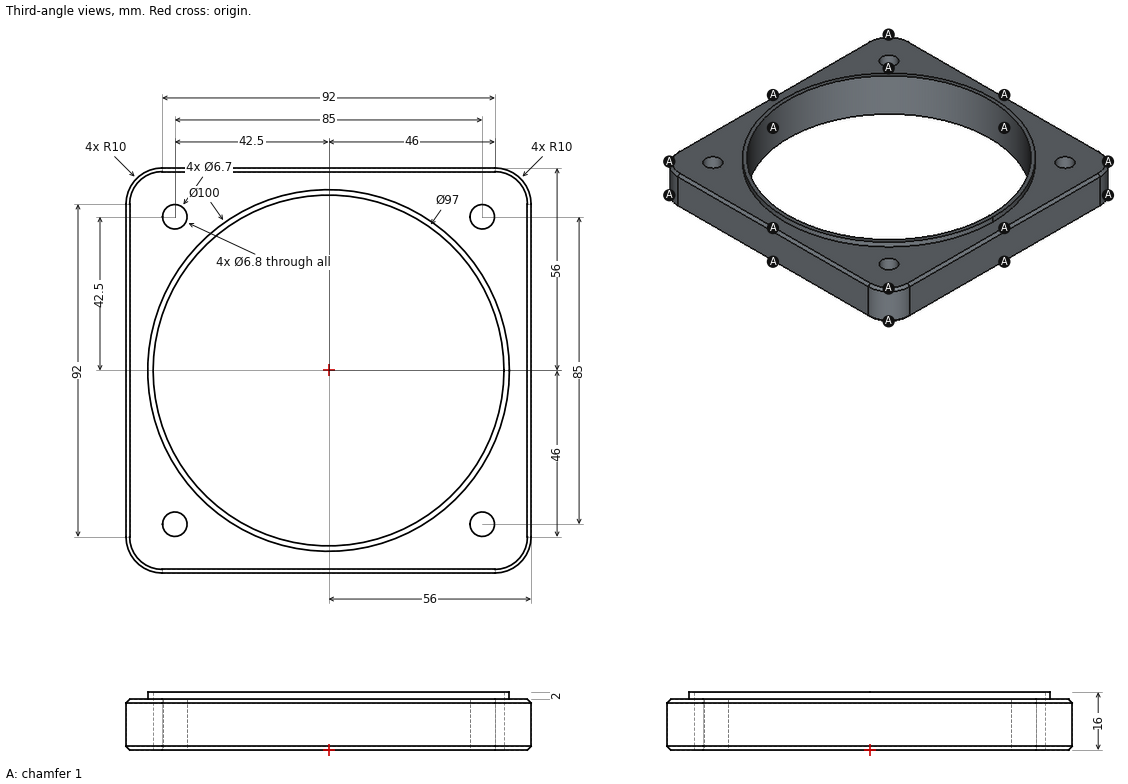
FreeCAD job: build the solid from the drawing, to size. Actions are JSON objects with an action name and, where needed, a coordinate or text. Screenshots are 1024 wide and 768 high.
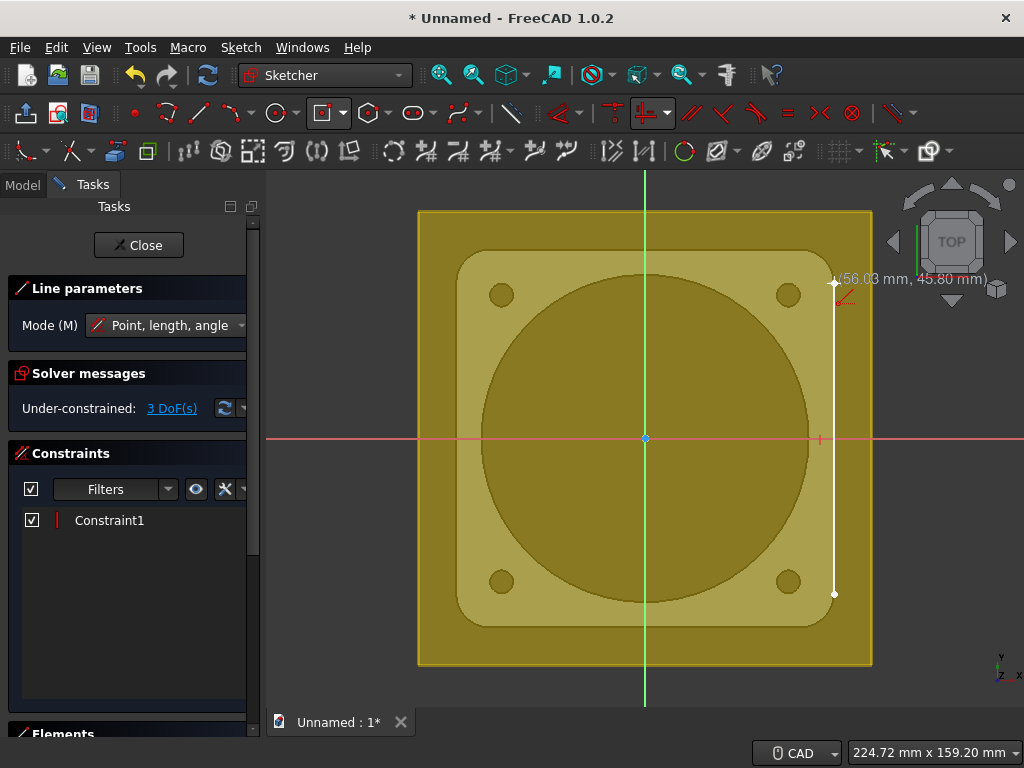
{"action": "left_click", "coordinate": [800, 250]}
{"action": "left_click", "coordinate": [490, 250]}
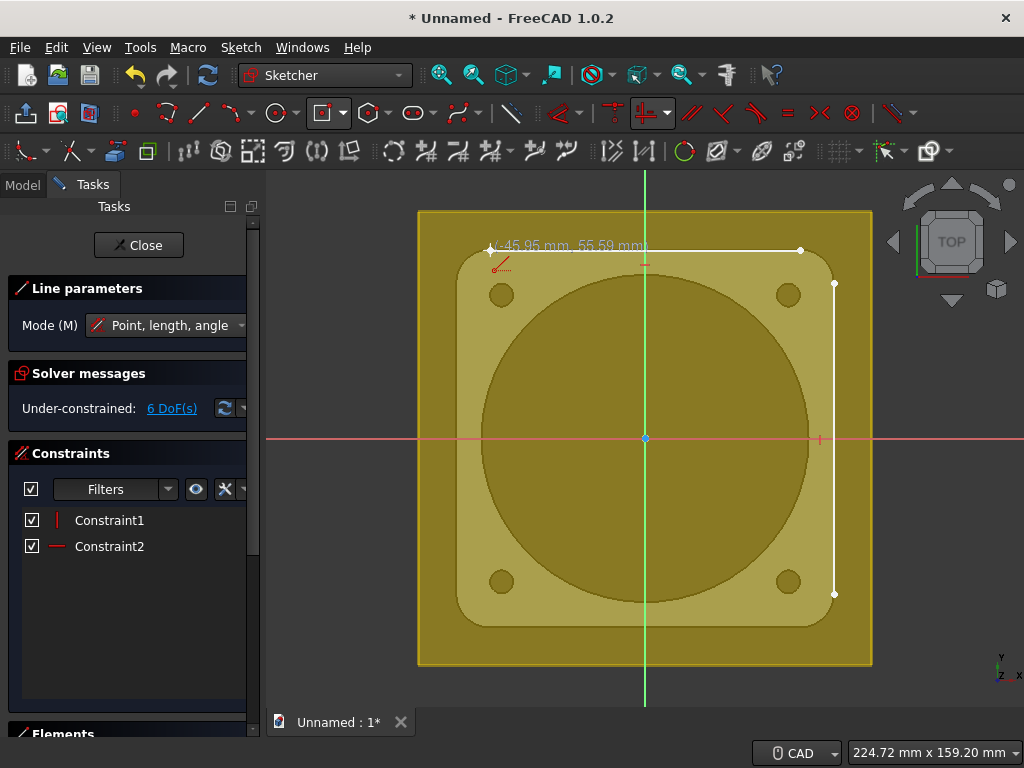
{"action": "left_click", "coordinate": [456, 283]}
{"action": "left_click", "coordinate": [456, 594]}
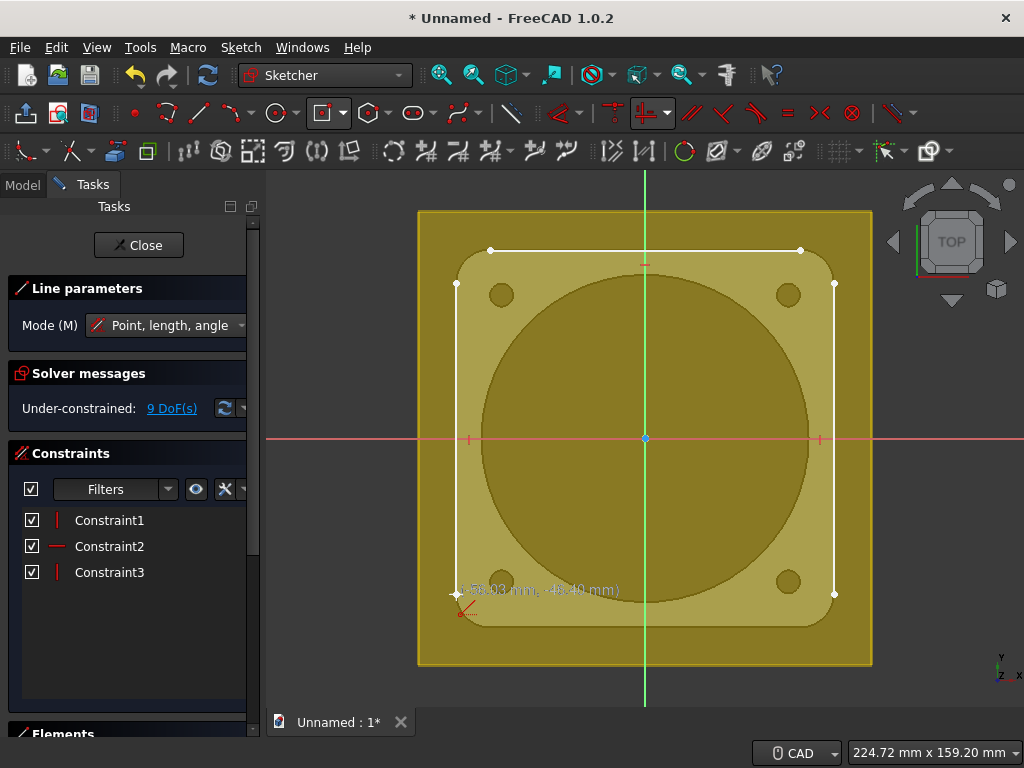
{"action": "left_click", "coordinate": [490, 627]}
{"action": "left_click", "coordinate": [800, 627]}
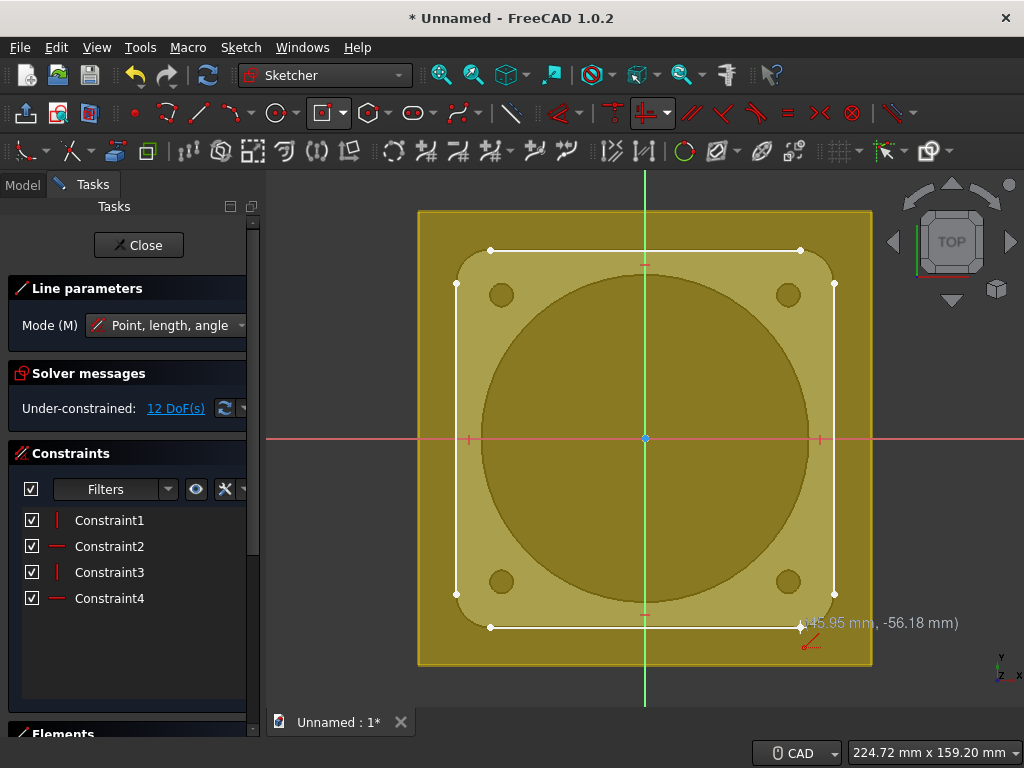
{"action": "left_click", "coordinate": [232, 114]}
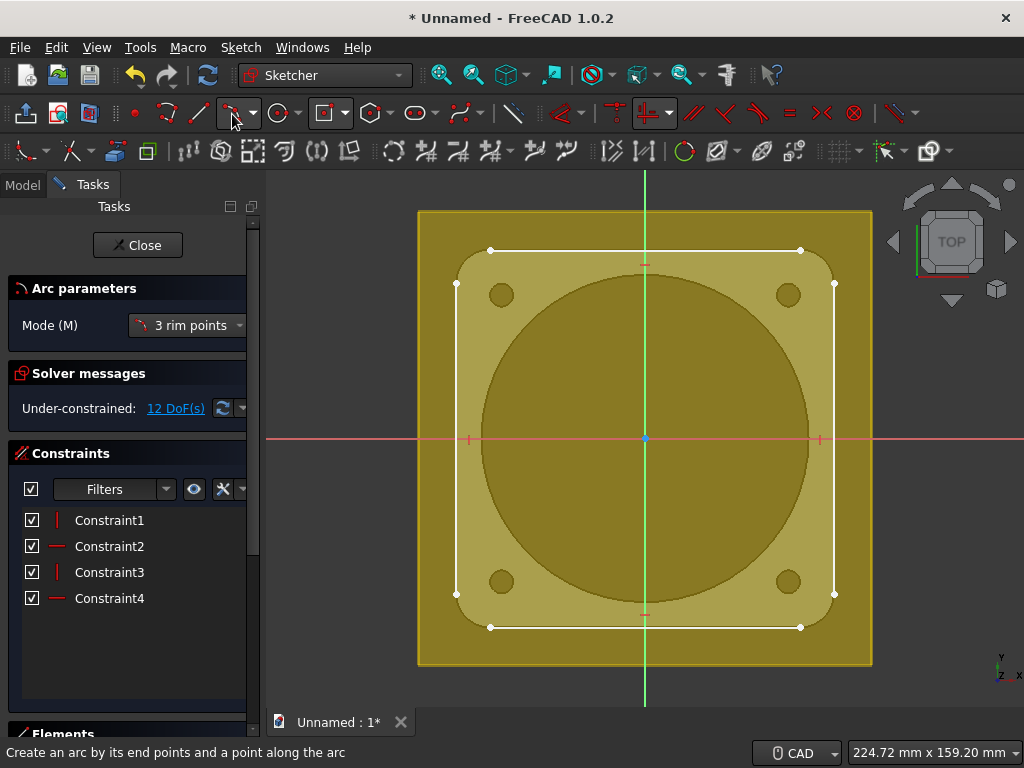
{"action": "left_click", "coordinate": [834, 284]}
{"action": "left_click", "coordinate": [800, 251]}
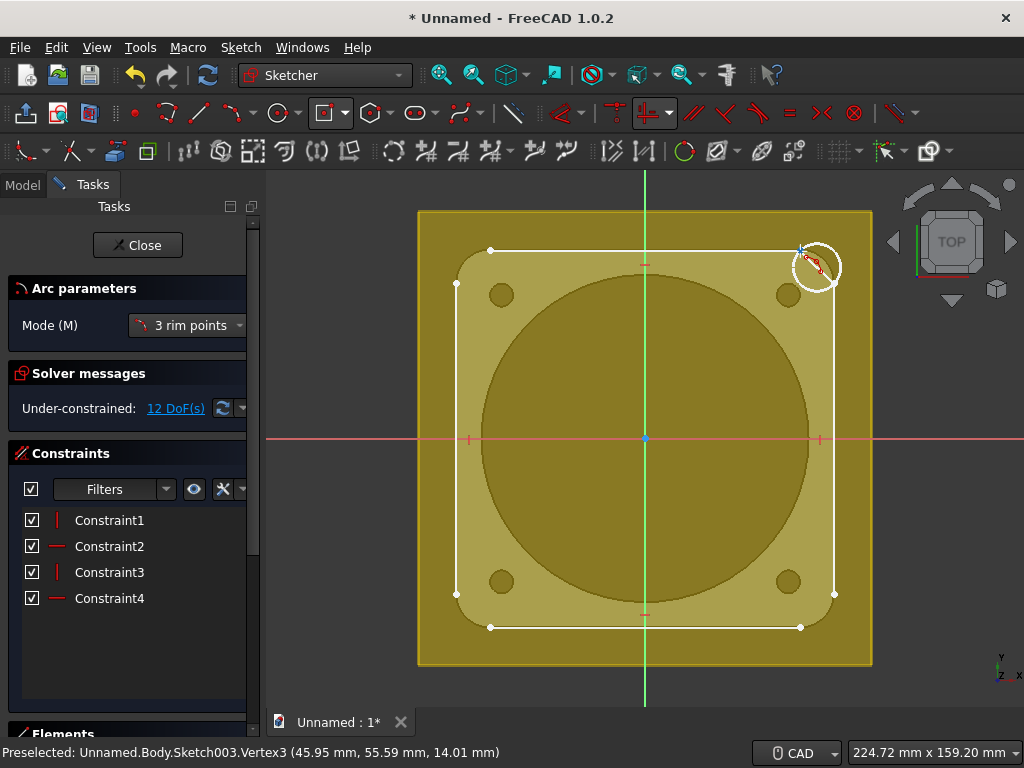
{"action": "scroll", "coordinate": [824, 259], "scroll_direction": "up", "scroll_amount": 3}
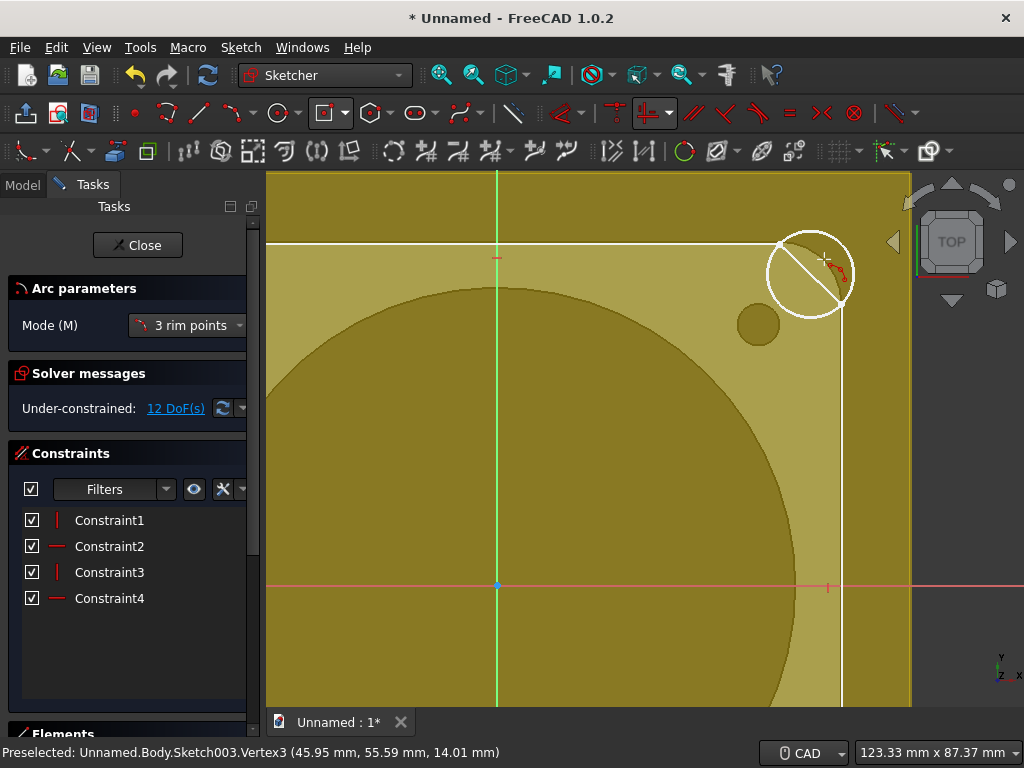
{"action": "left_click", "coordinate": [823, 260]}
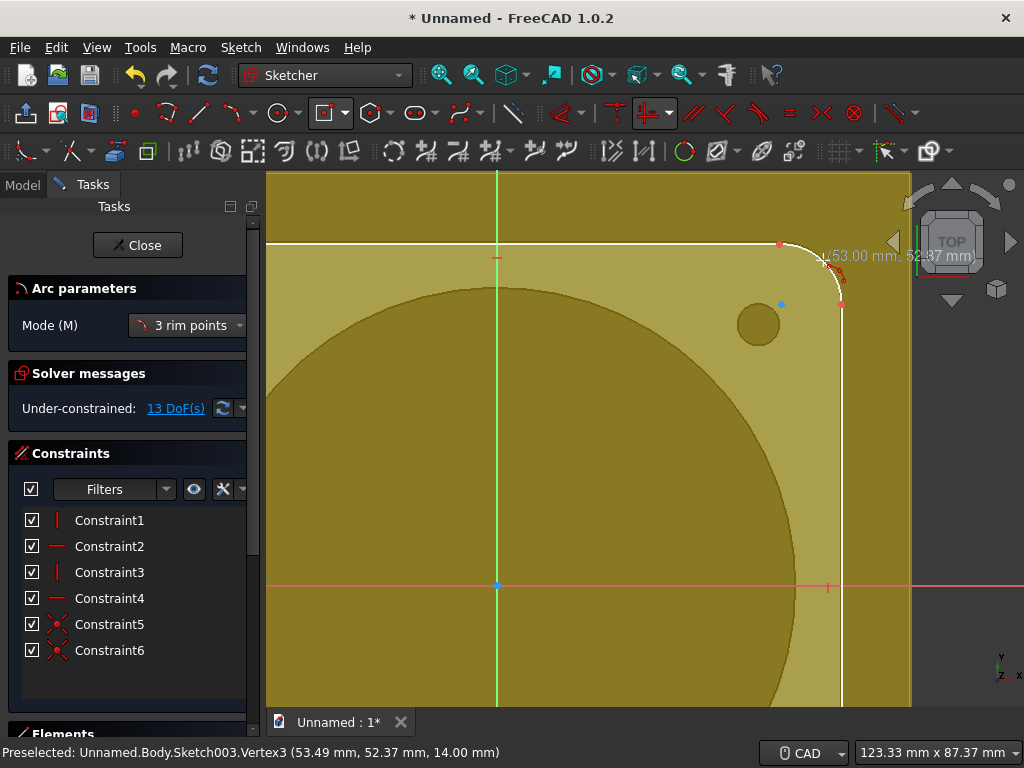
{"action": "scroll", "coordinate": [641, 318], "scroll_direction": "down", "scroll_amount": 4}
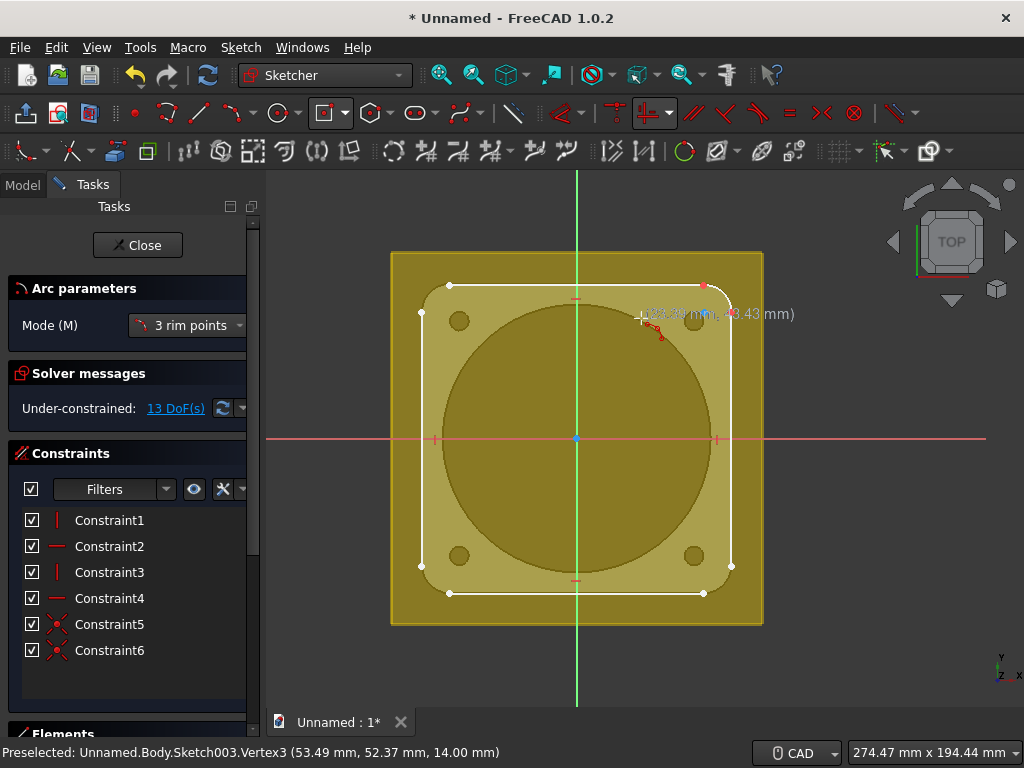
{"action": "left_click", "coordinate": [450, 285]}
{"action": "left_click", "coordinate": [422, 312]}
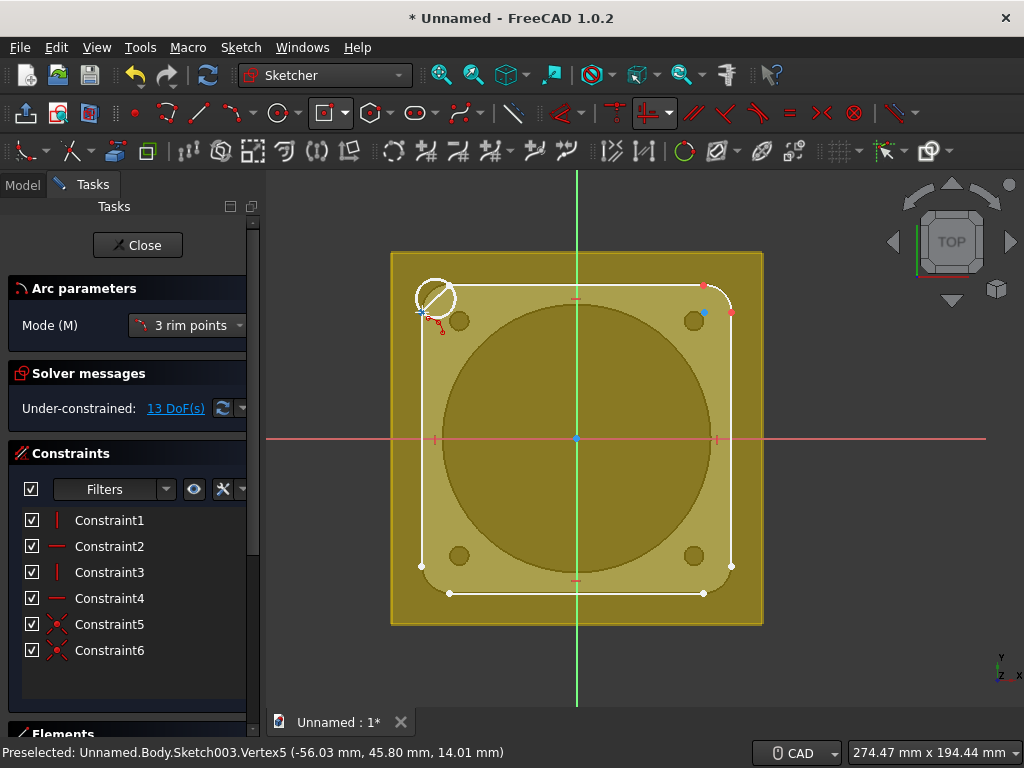
{"action": "scroll", "coordinate": [430, 292], "scroll_direction": "up", "scroll_amount": 4}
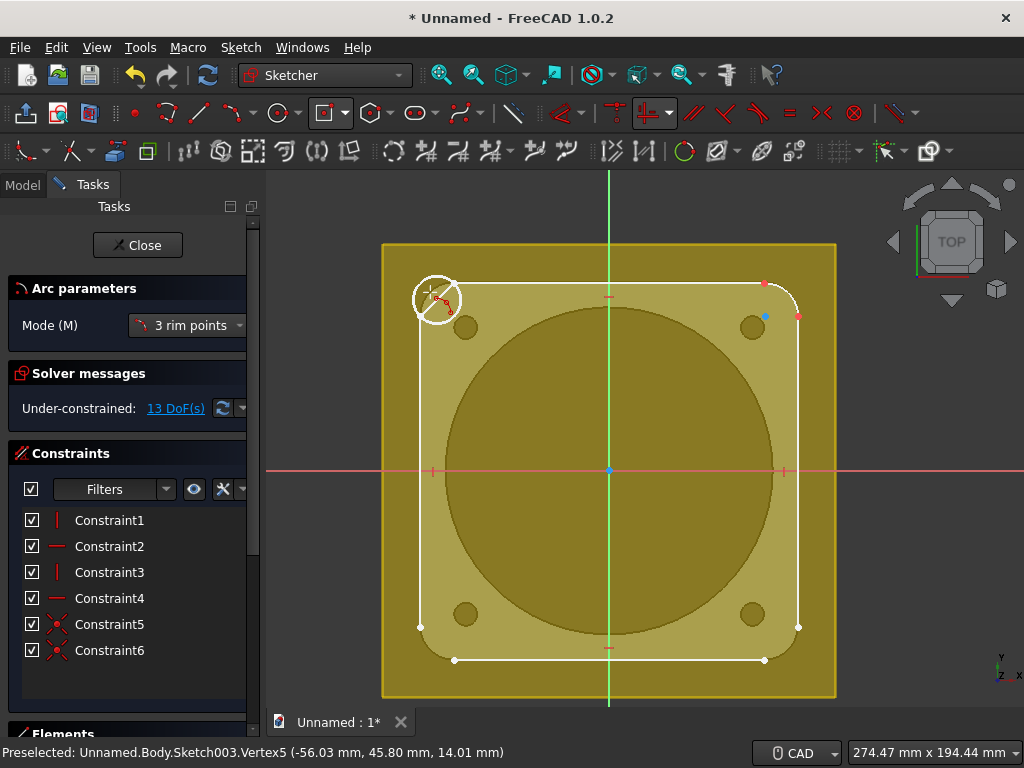
{"action": "left_click", "coordinate": [430, 292]}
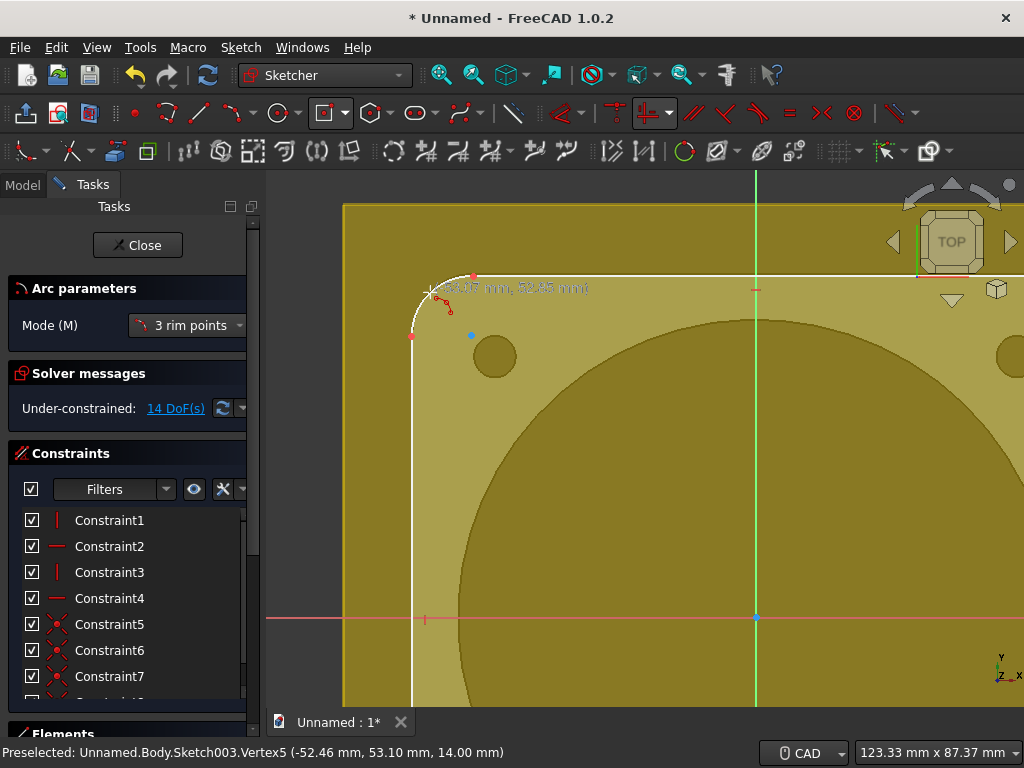
{"action": "scroll", "coordinate": [430, 292], "scroll_direction": "down", "scroll_amount": 4}